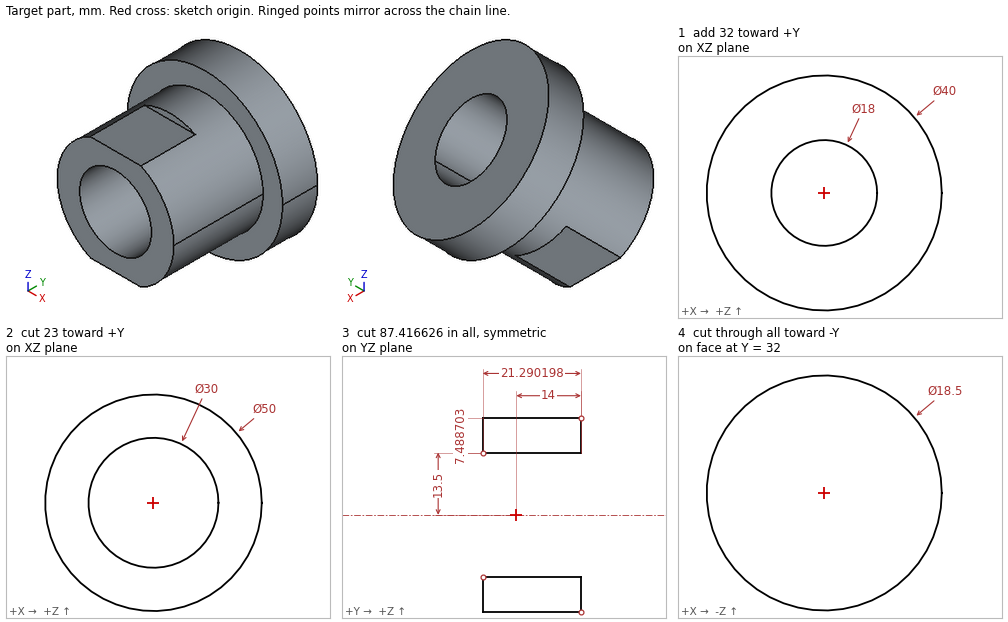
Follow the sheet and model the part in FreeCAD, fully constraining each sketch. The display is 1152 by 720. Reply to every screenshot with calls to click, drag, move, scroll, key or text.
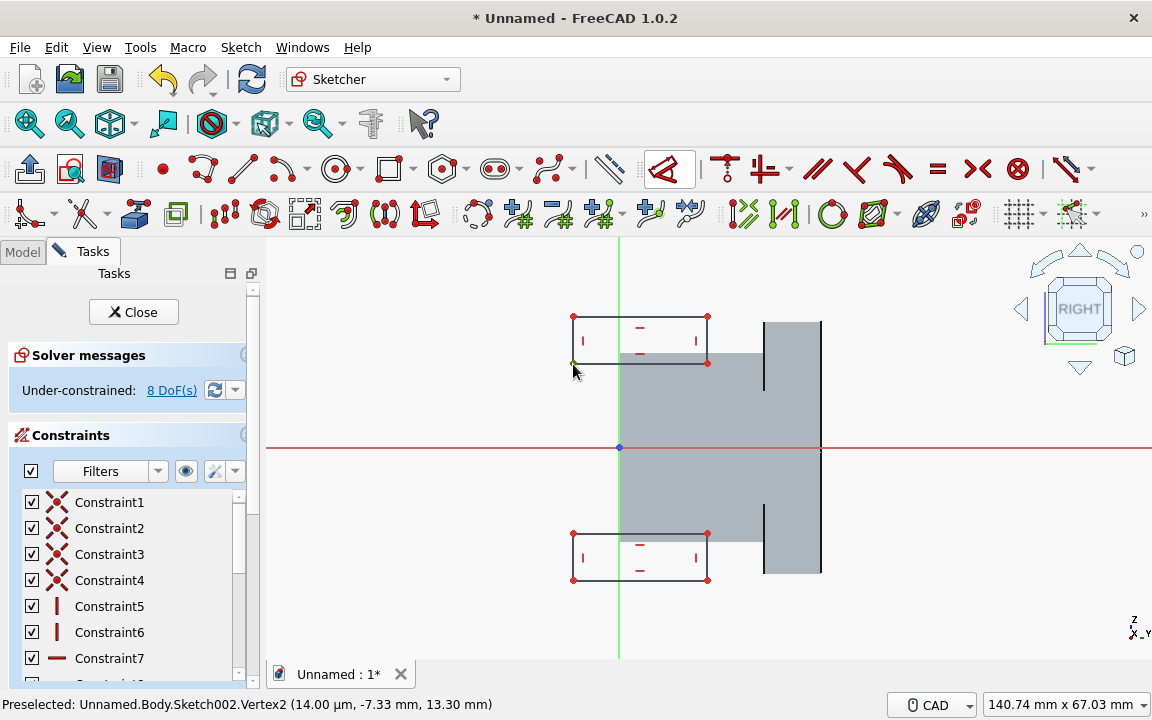
click(573, 534)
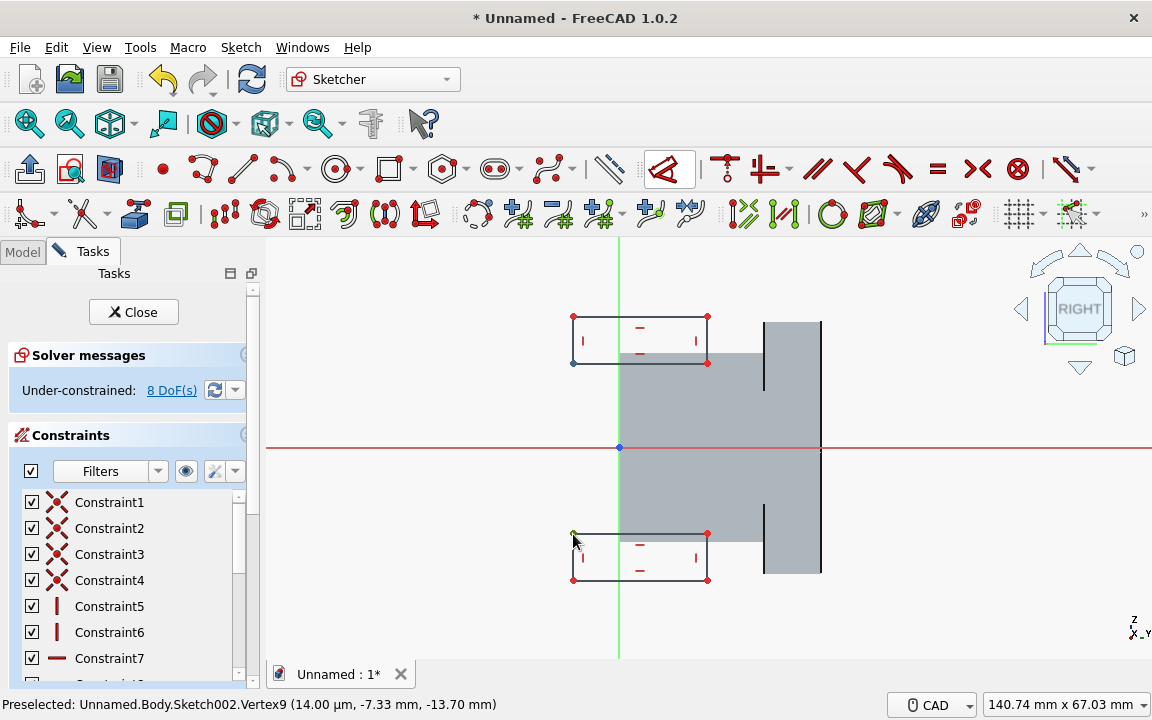
click(344, 448)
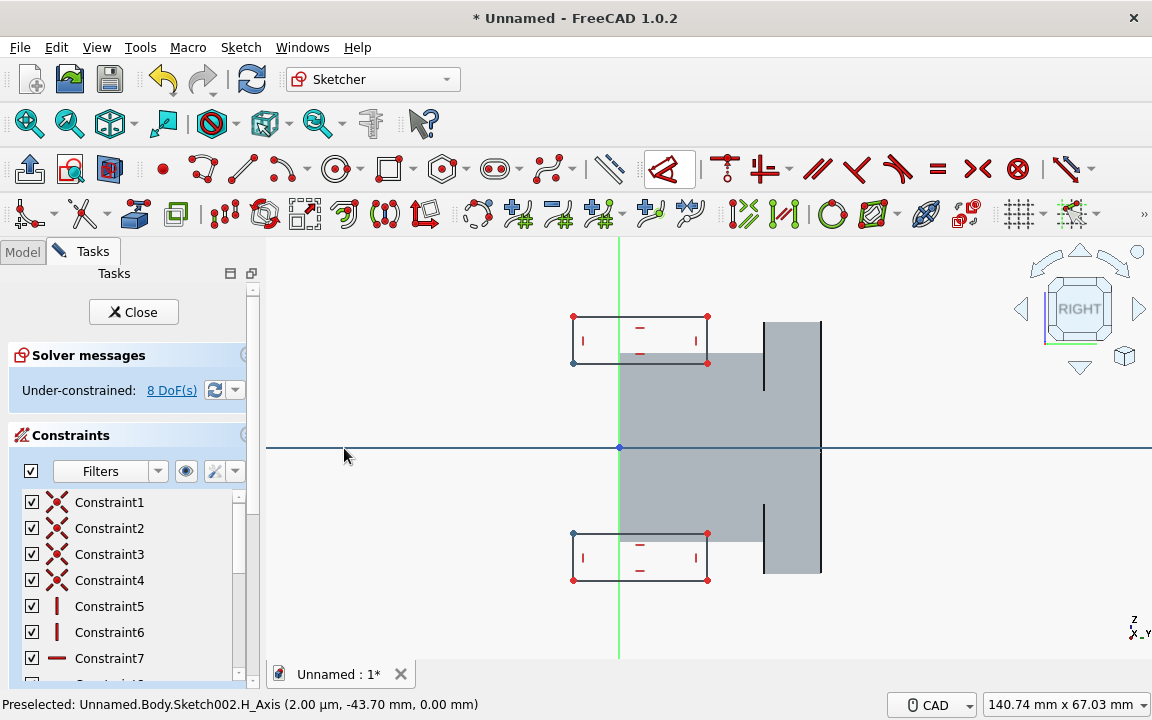
click(978, 170)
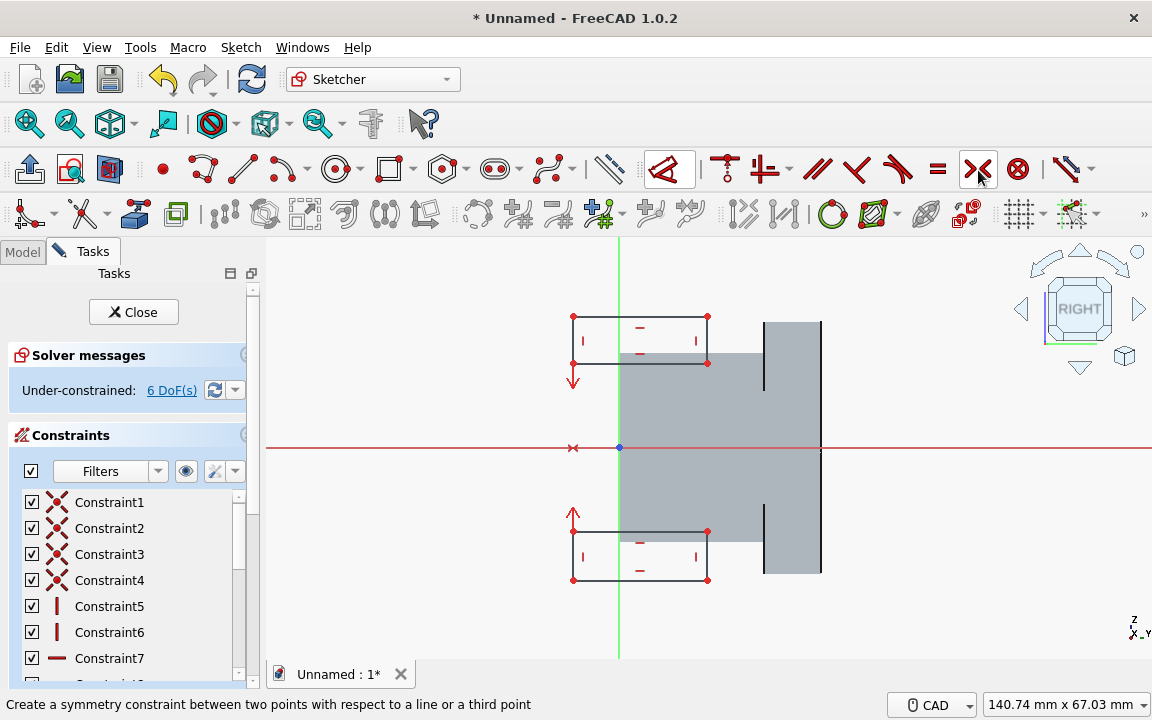
click(707, 317)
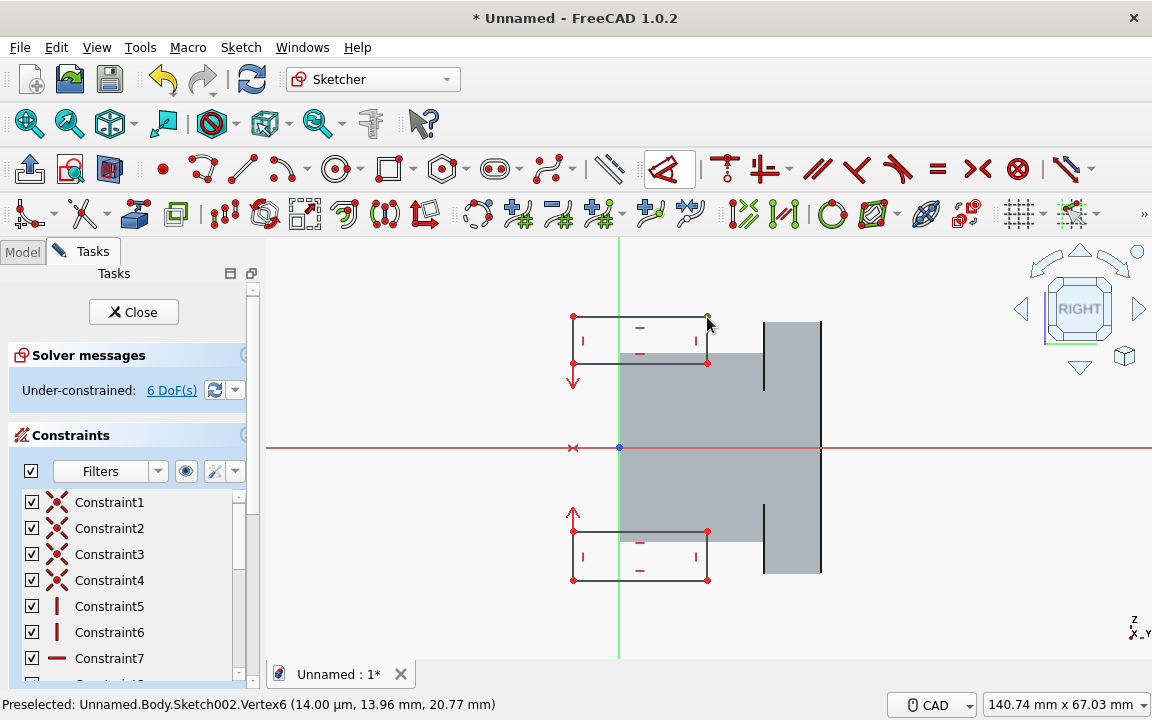
click(707, 581)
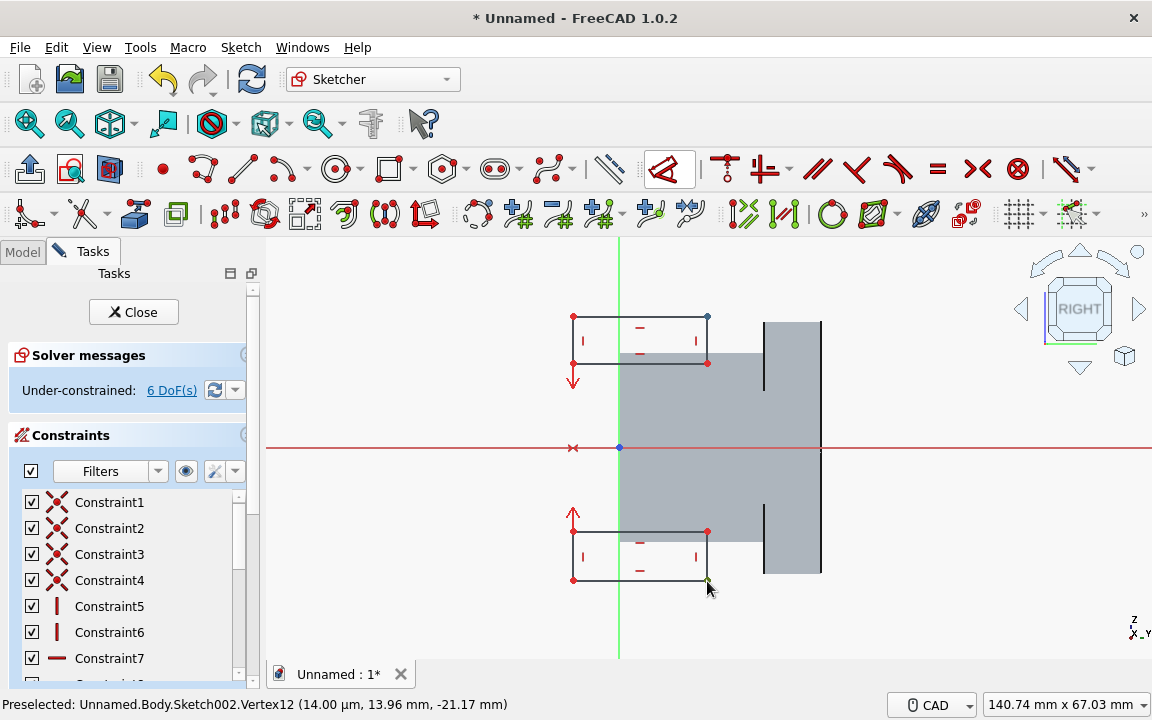
click(344, 448)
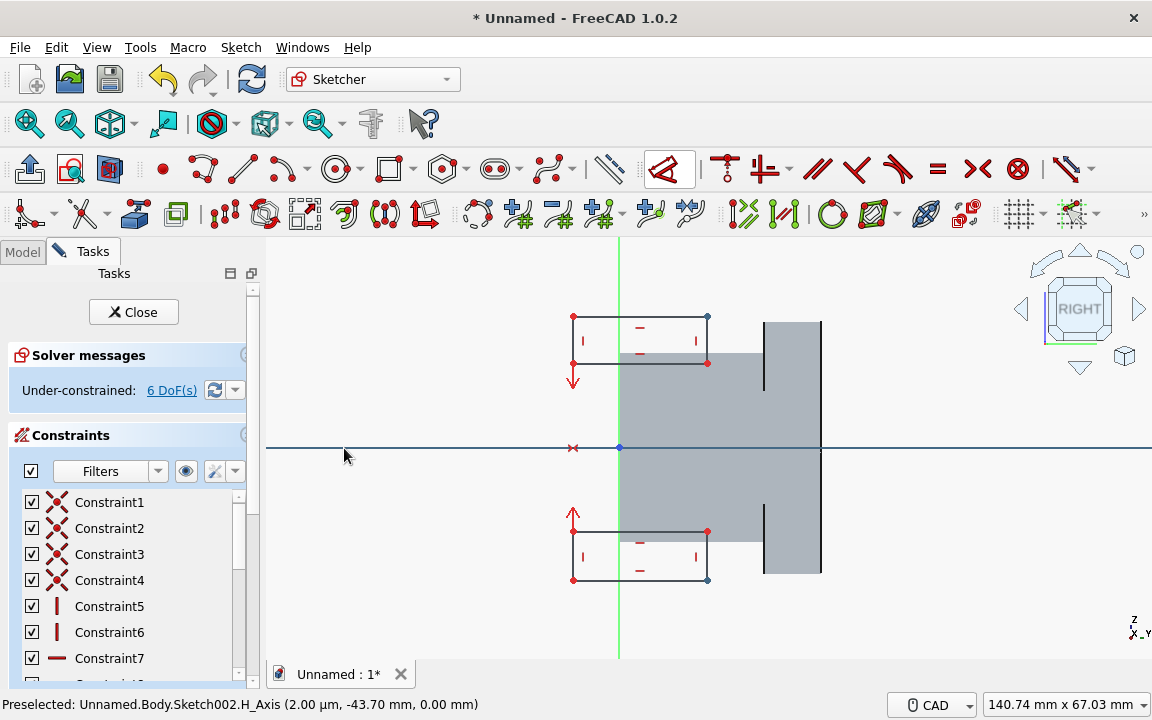
key(s)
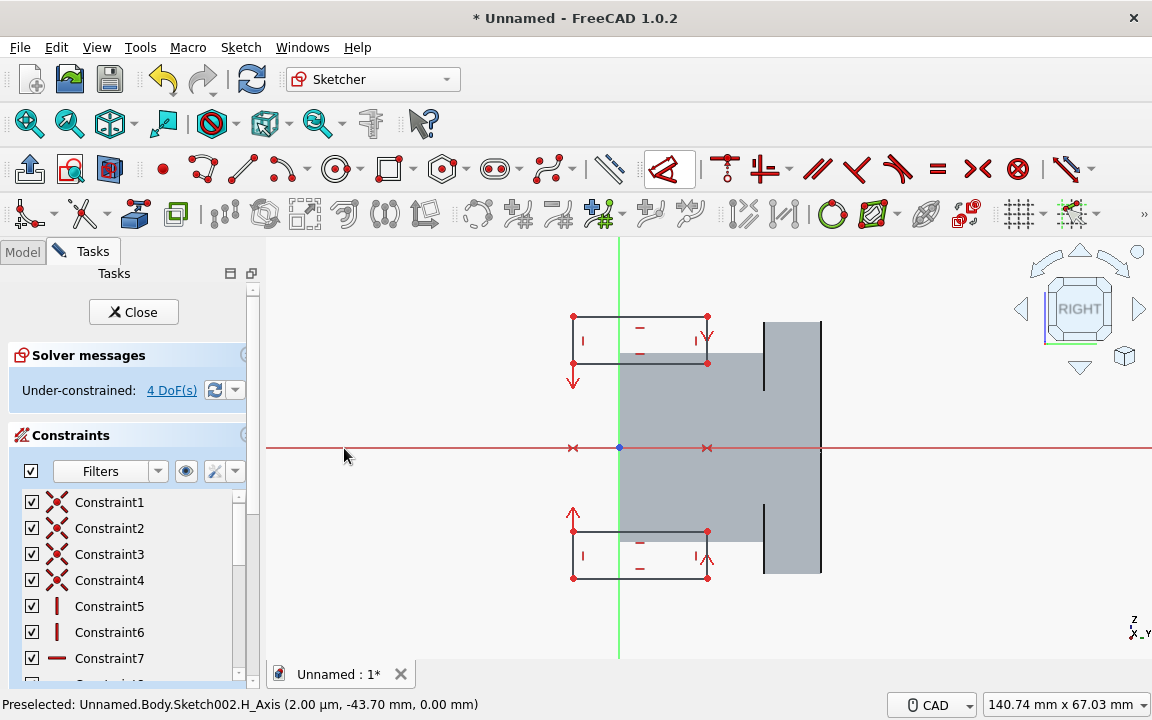
click(707, 364)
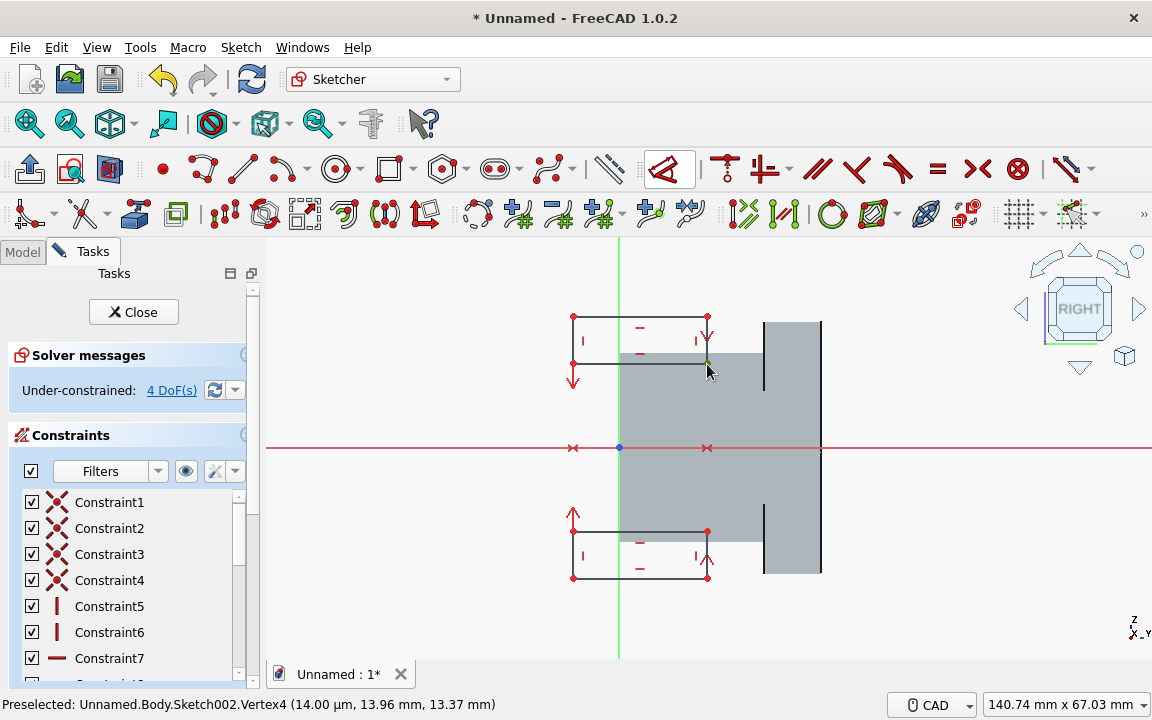
click(690, 170)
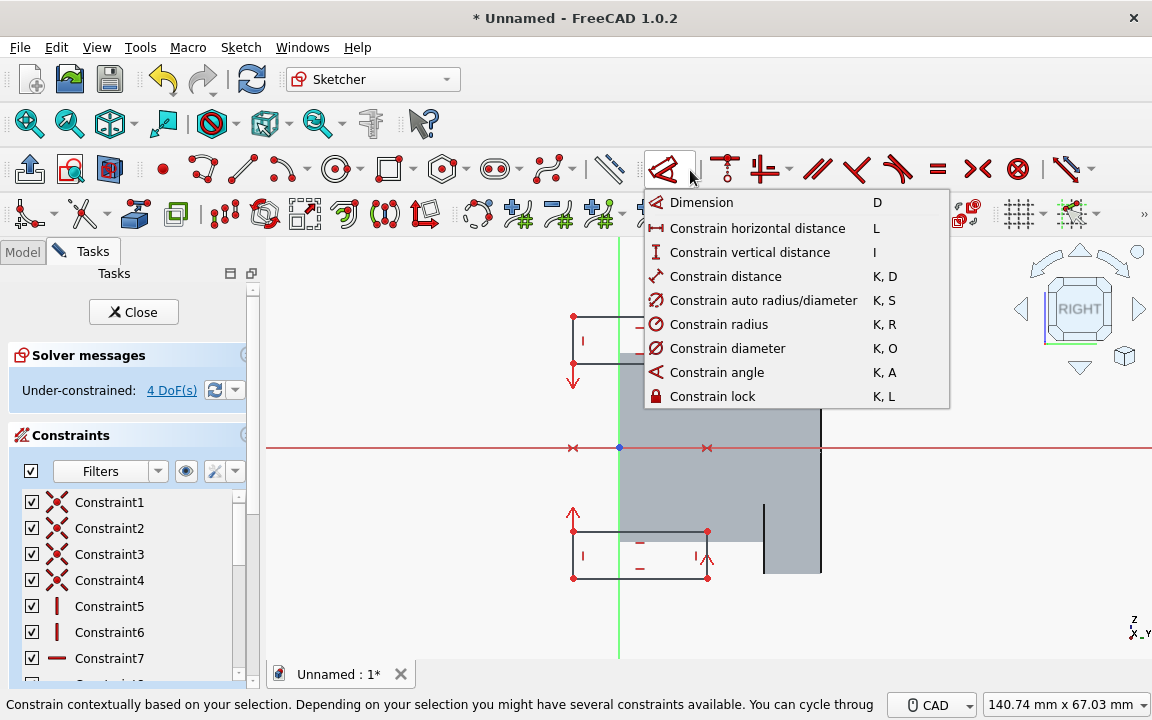
click(797, 228)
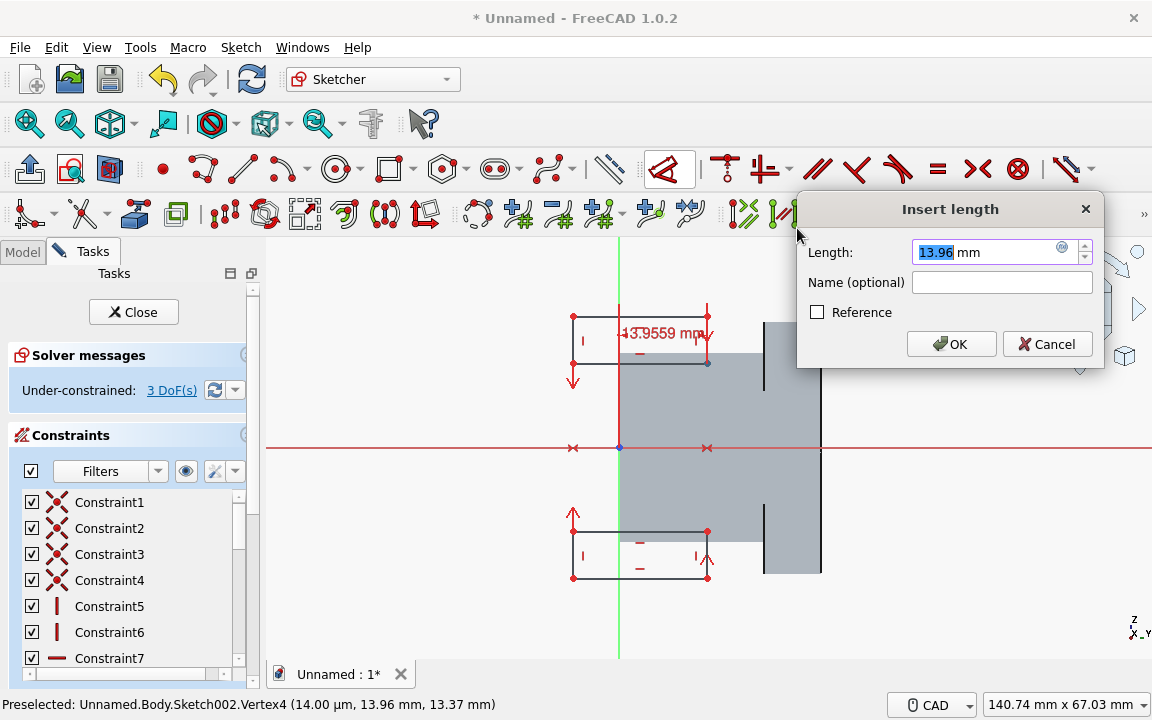
text(14)
key(Return)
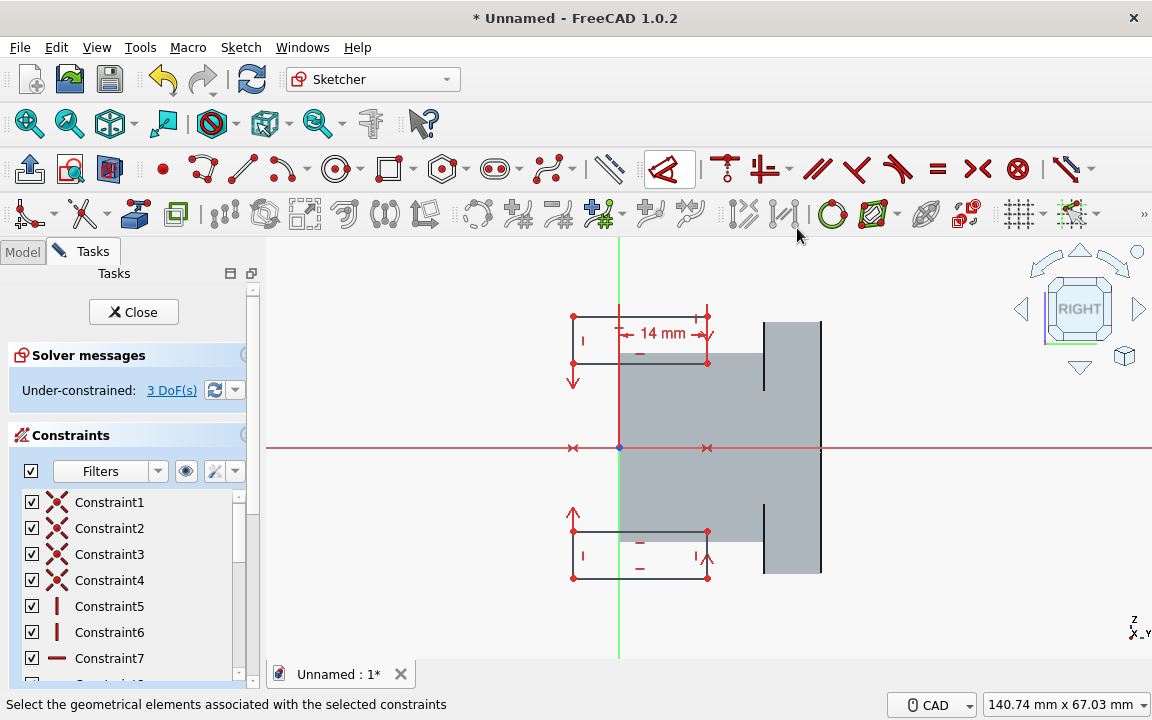
click(573, 364)